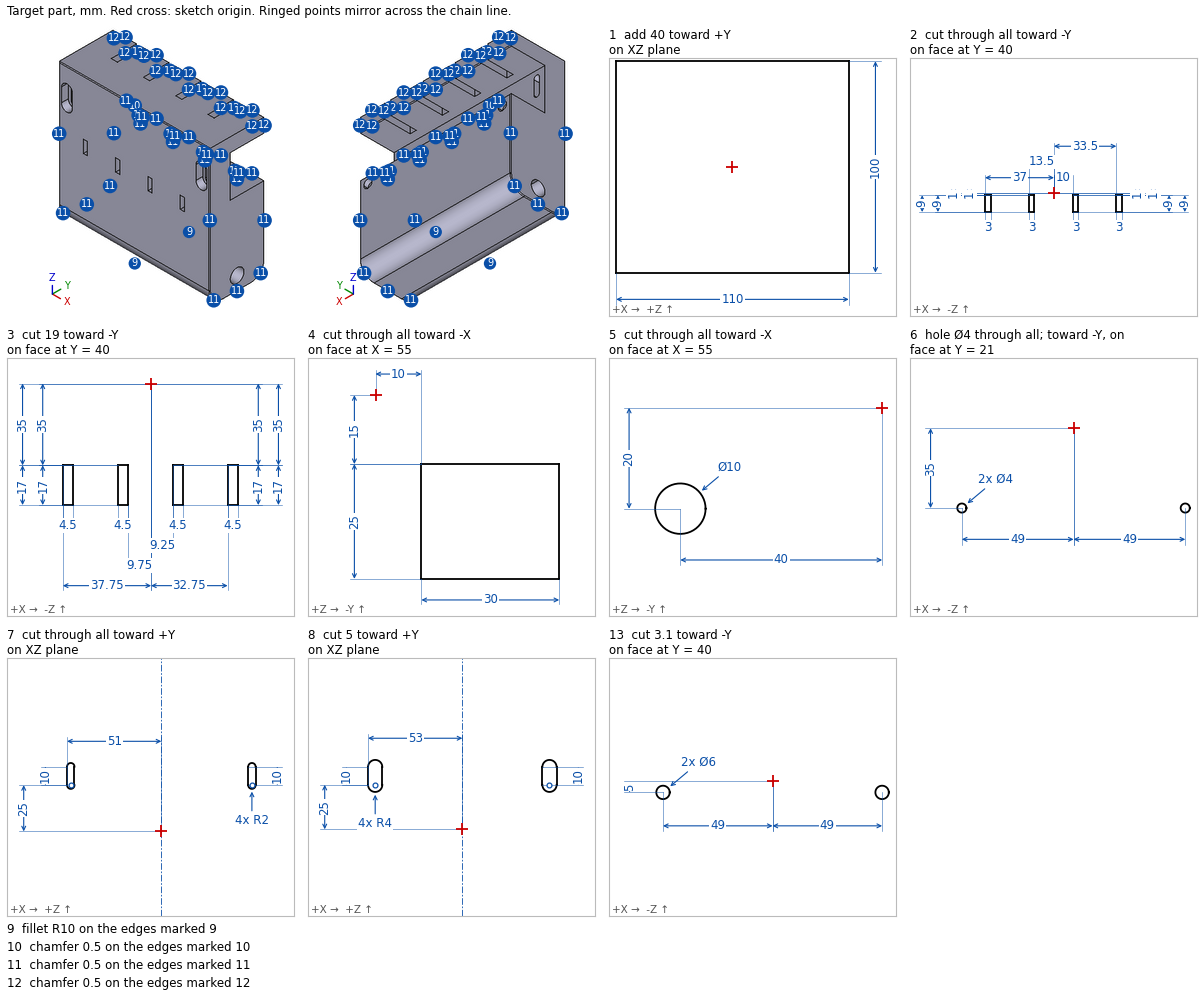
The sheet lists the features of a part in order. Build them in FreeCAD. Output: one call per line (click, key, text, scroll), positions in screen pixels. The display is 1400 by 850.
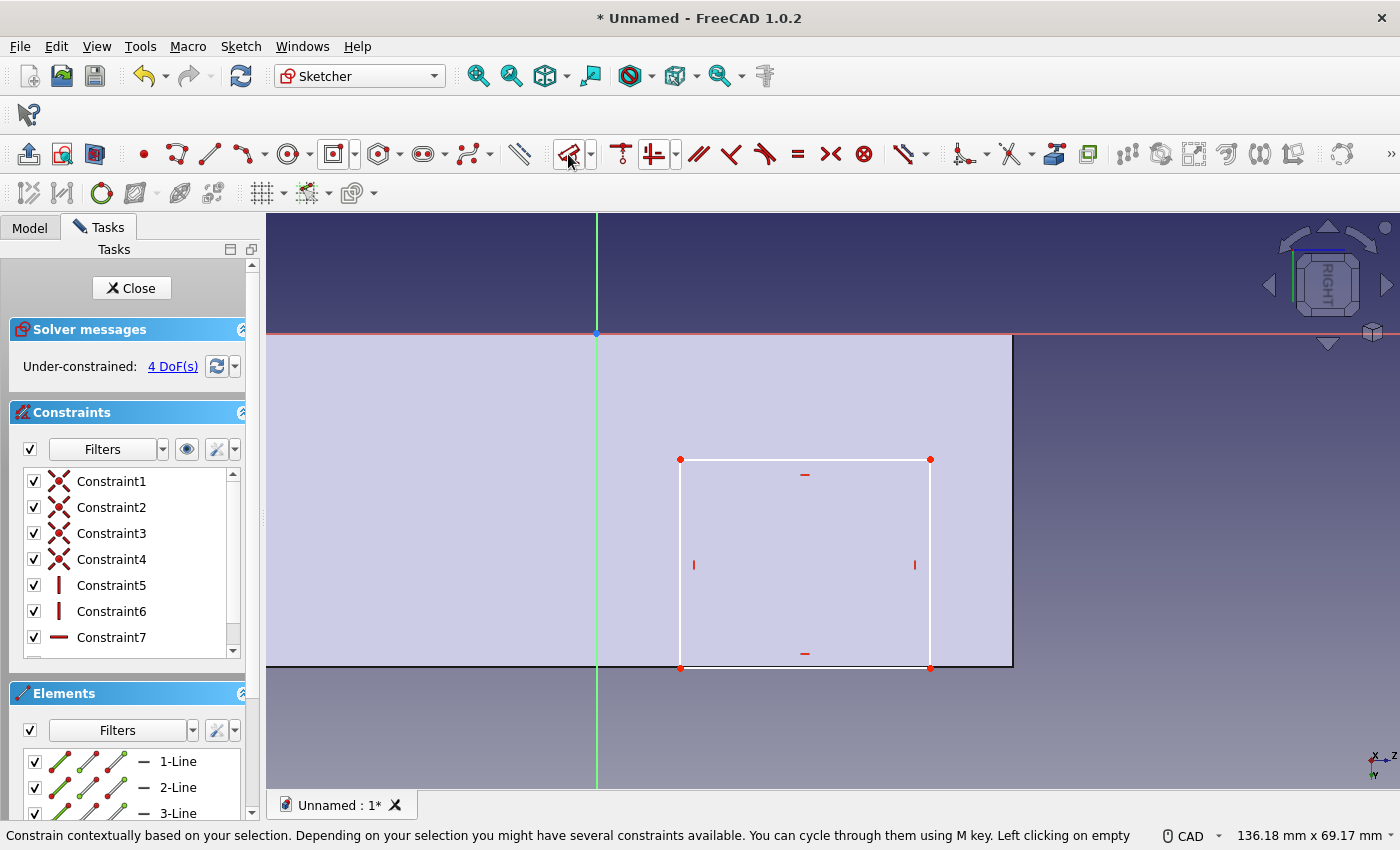
click(680, 522)
click(646, 564)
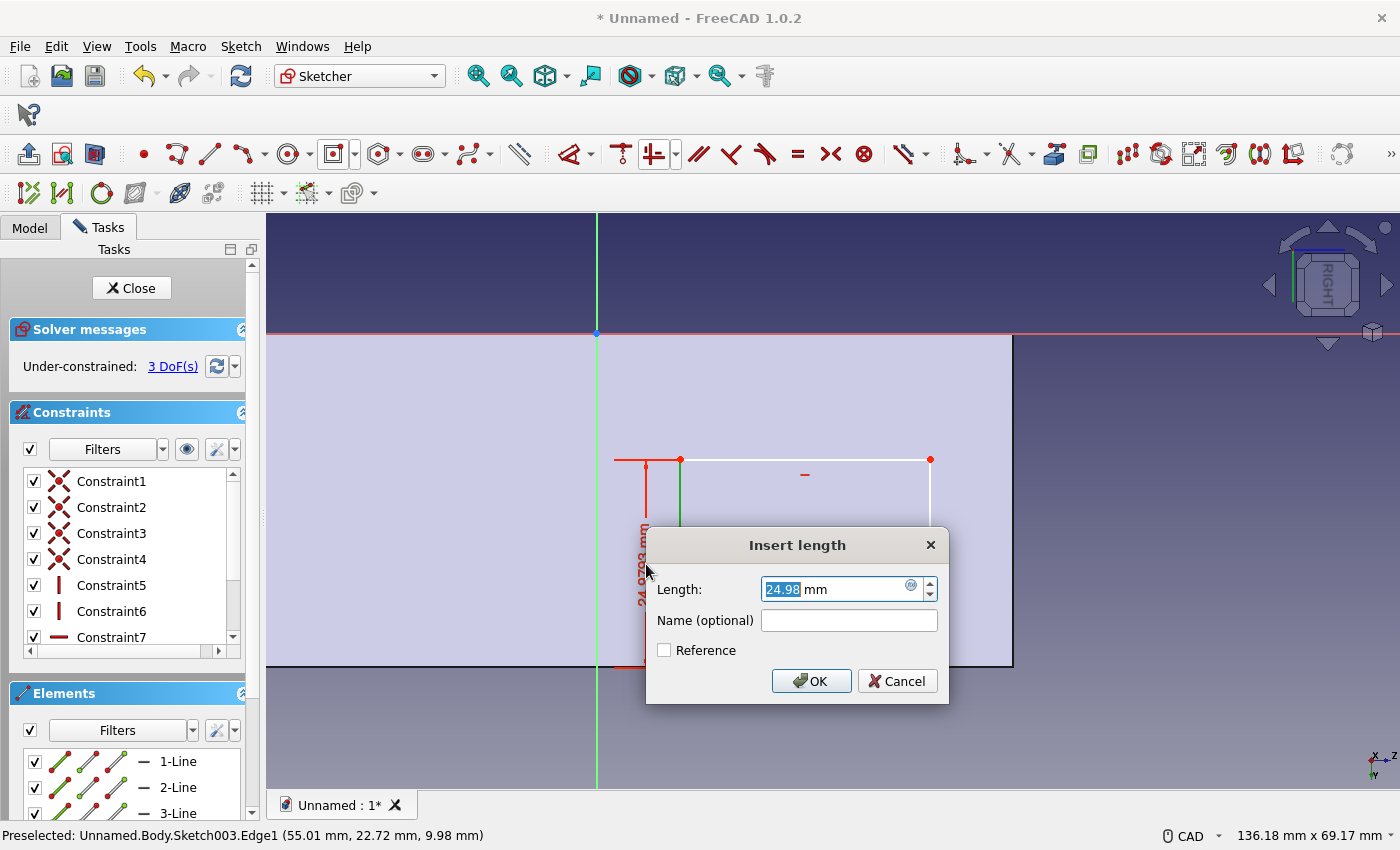
text(25)
key(Return)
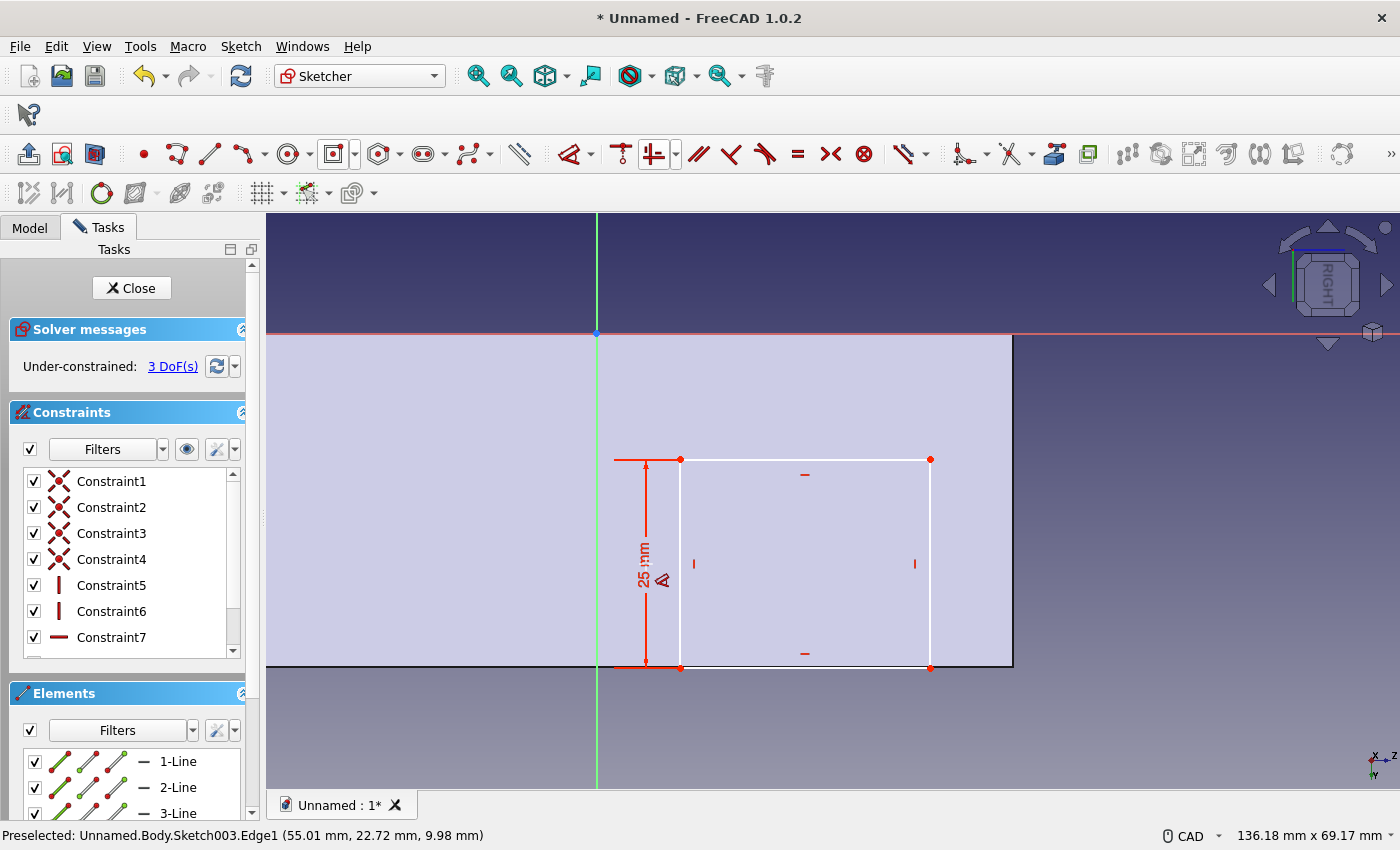
click(755, 668)
click(805, 702)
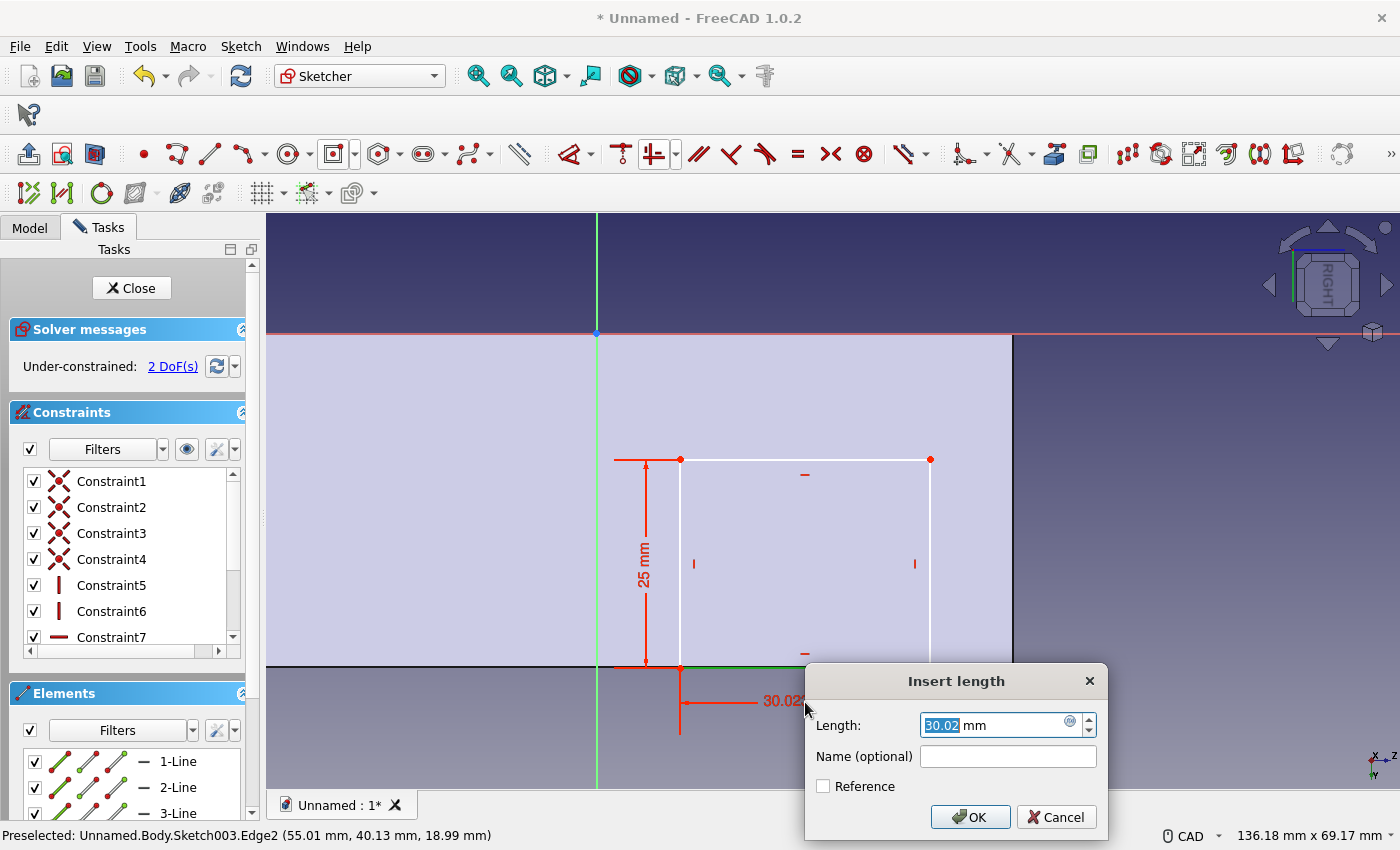
text(30)
key(Return)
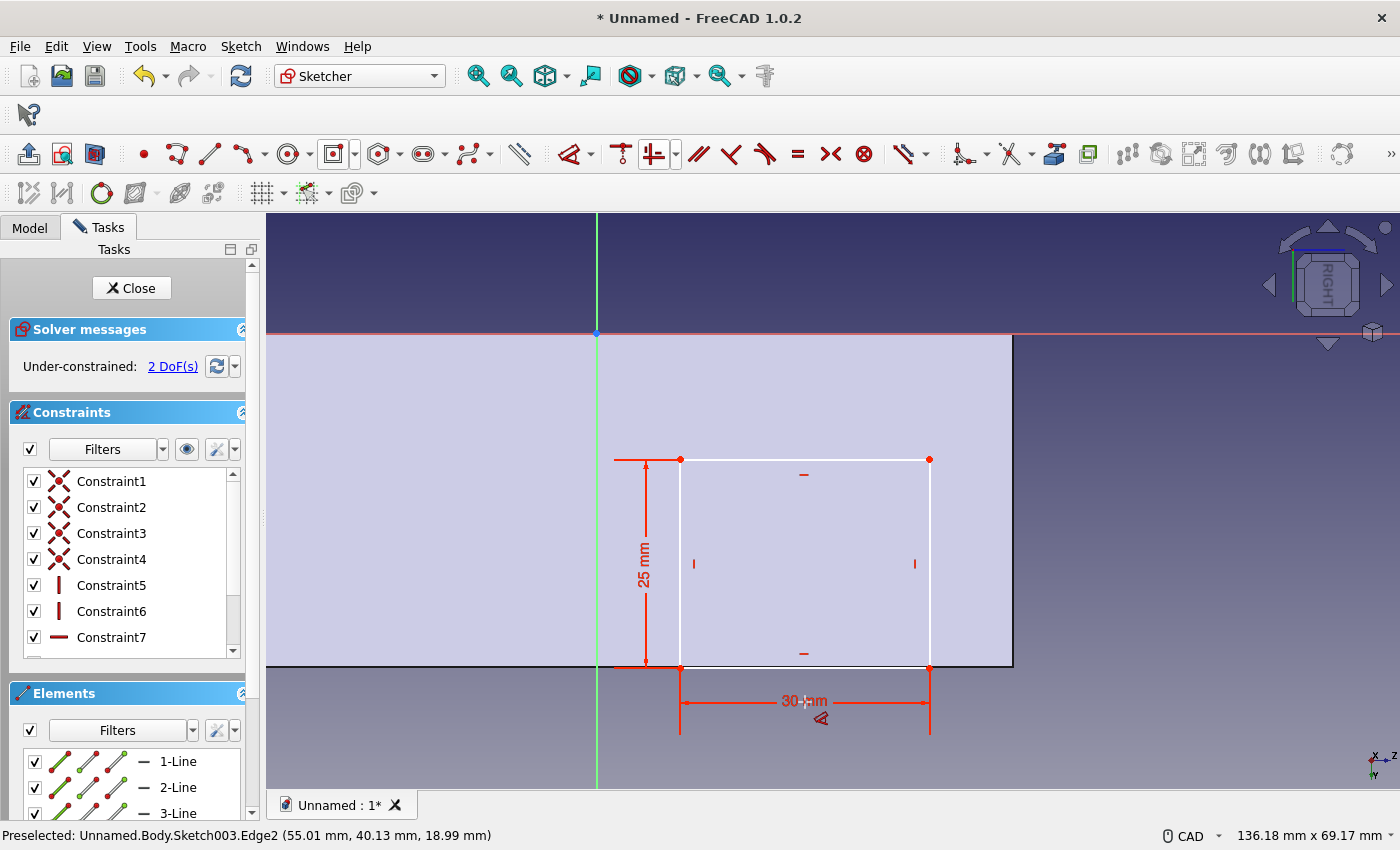
click(680, 460)
click(638, 300)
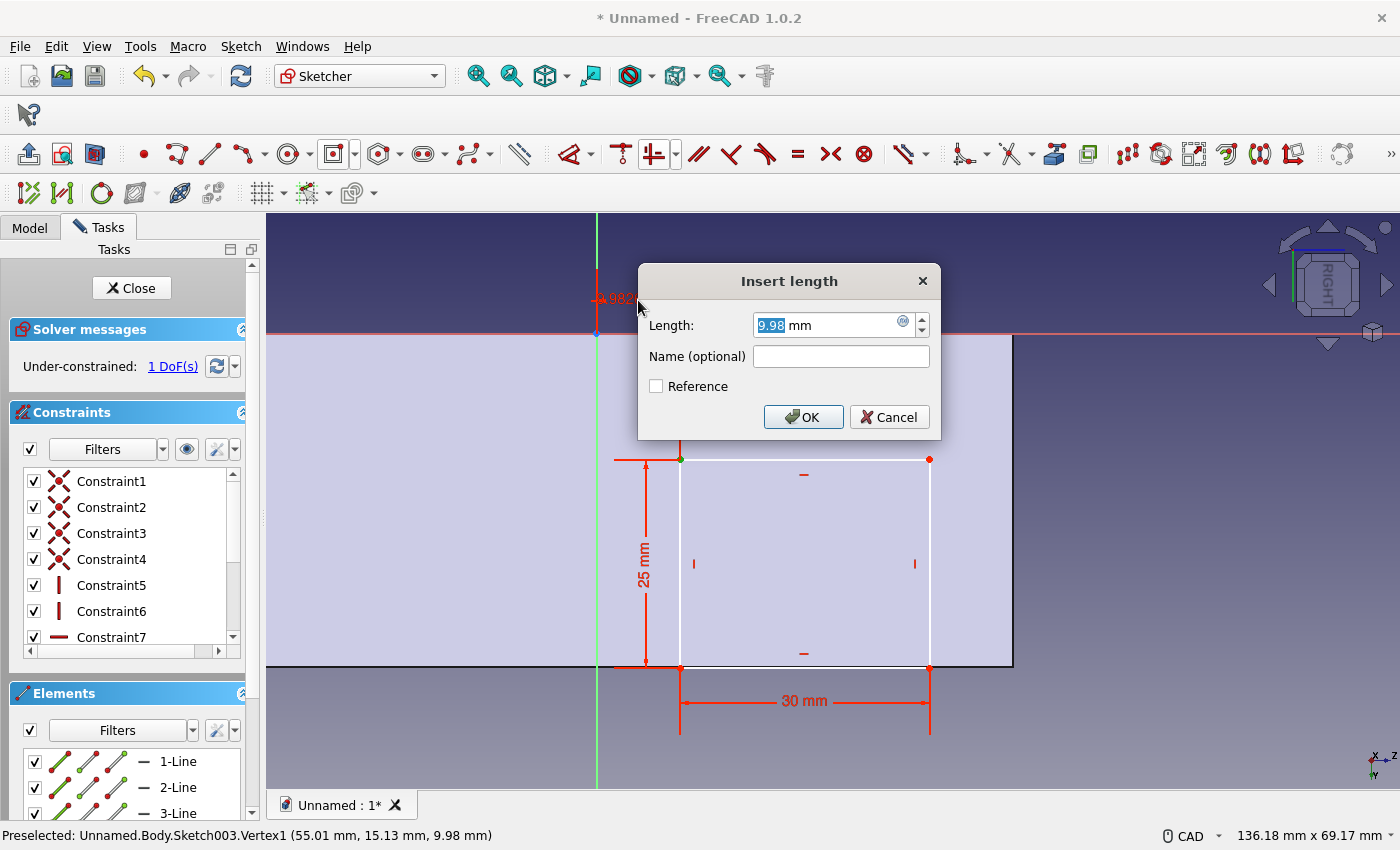
text(10)
key(Return)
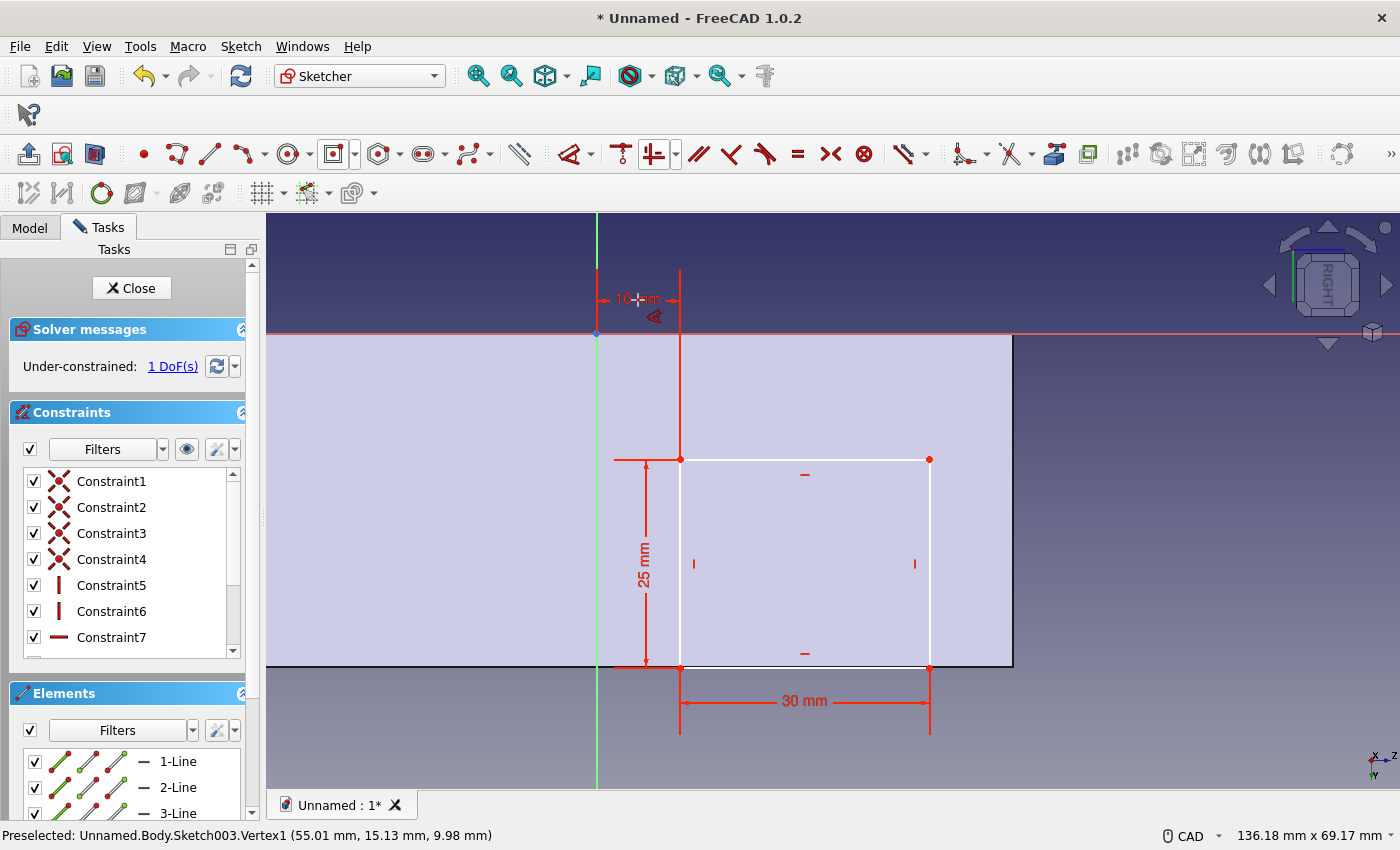
click(680, 460)
click(563, 397)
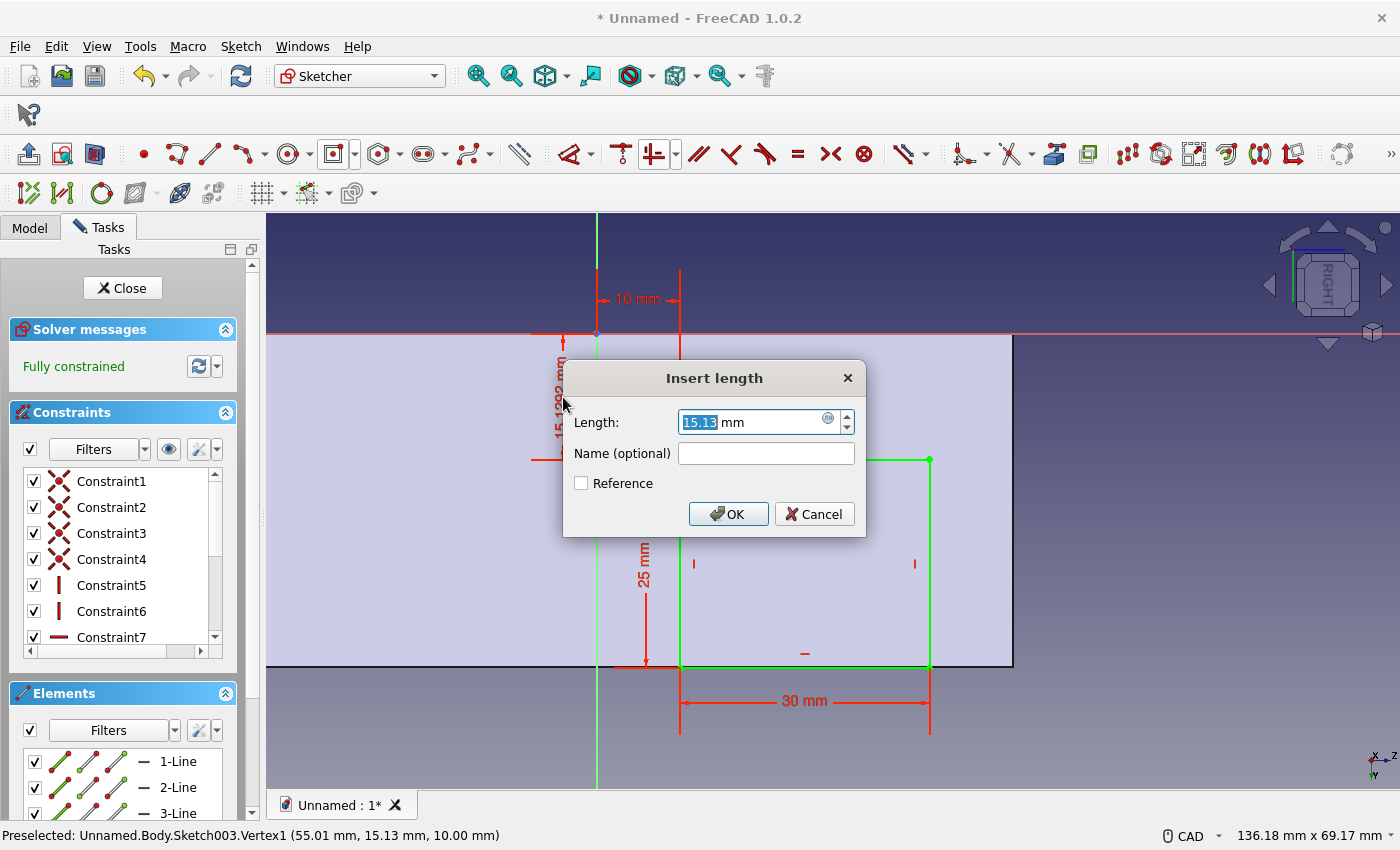
text(15)
key(Return)
key(Escape)